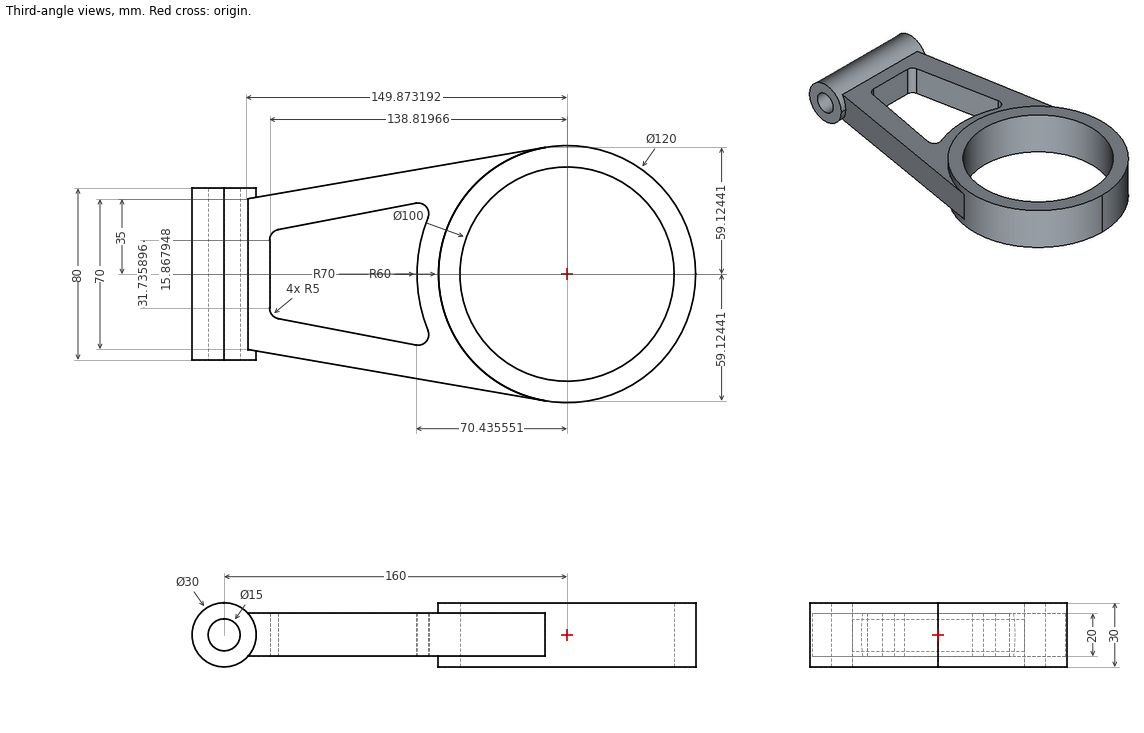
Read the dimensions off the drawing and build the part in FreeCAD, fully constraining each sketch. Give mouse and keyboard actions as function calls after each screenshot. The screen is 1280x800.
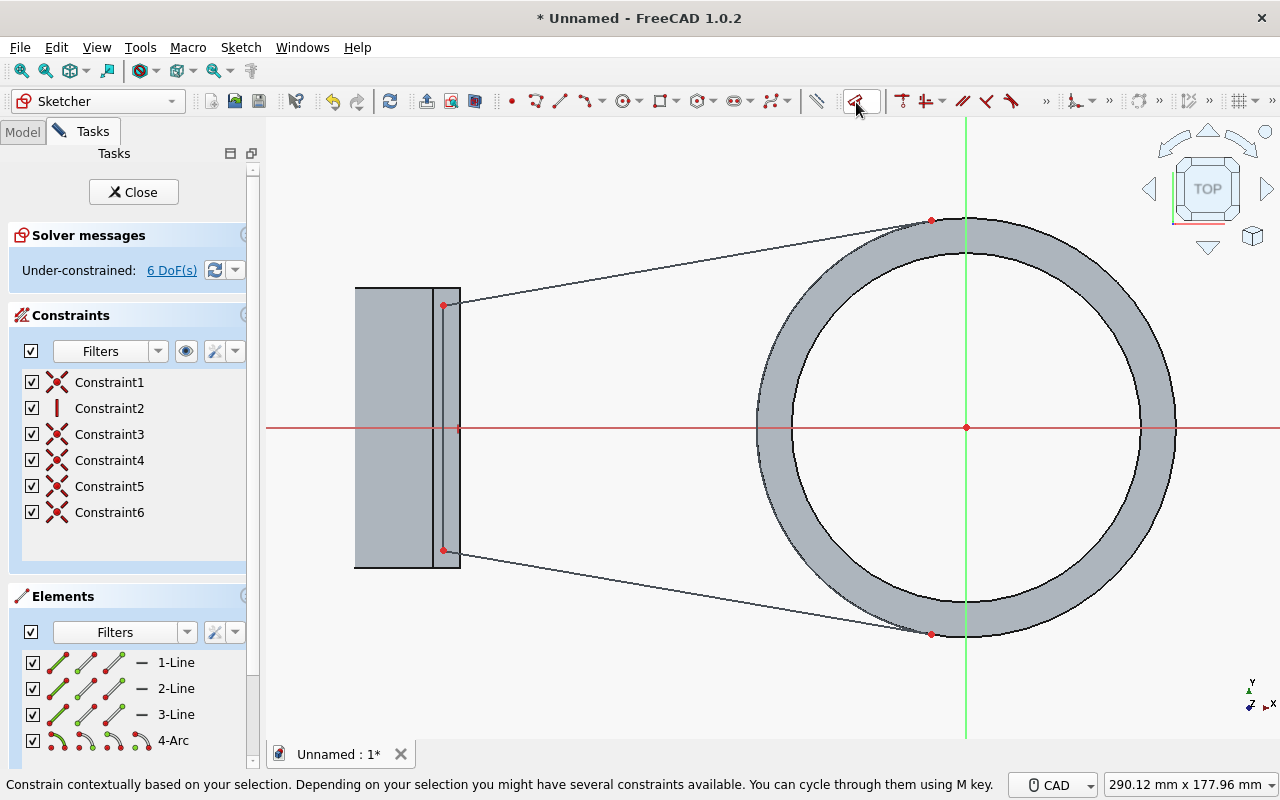
click(789, 316)
click(762, 299)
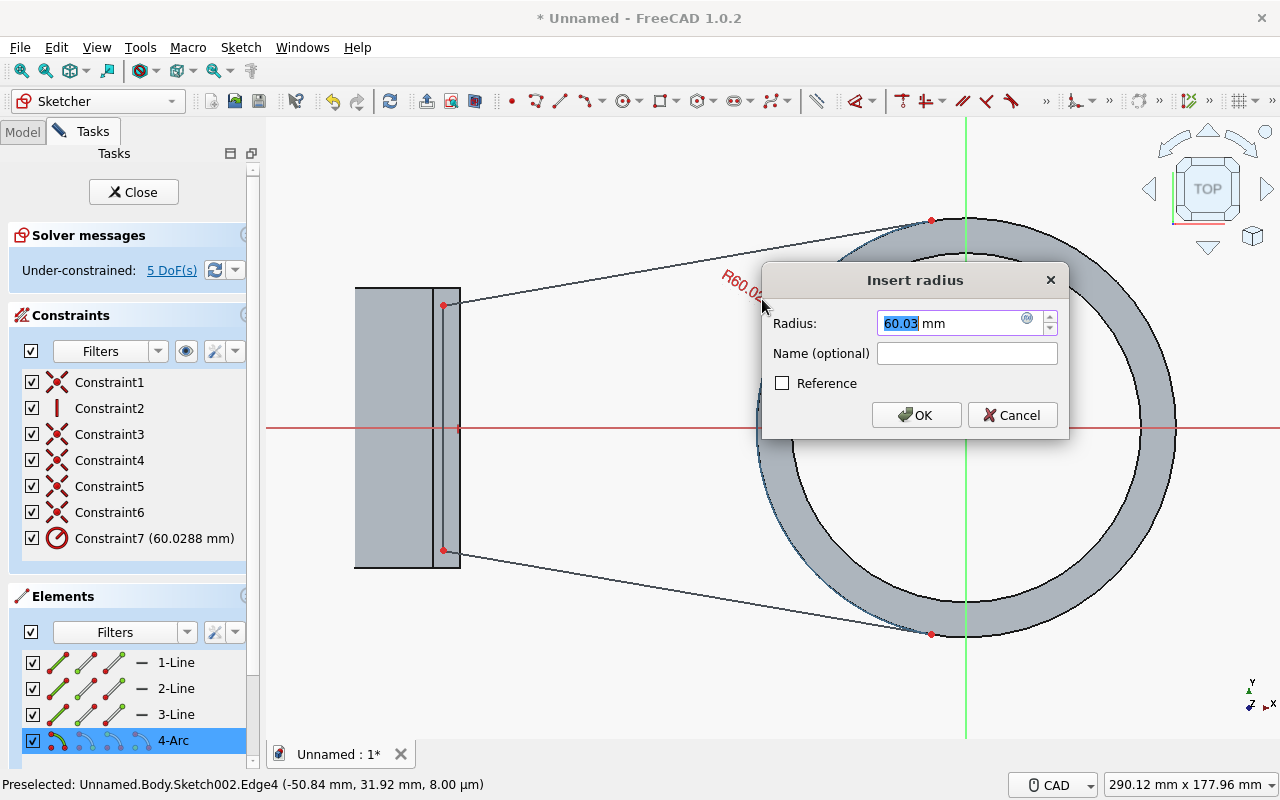
text(60)
key(Return)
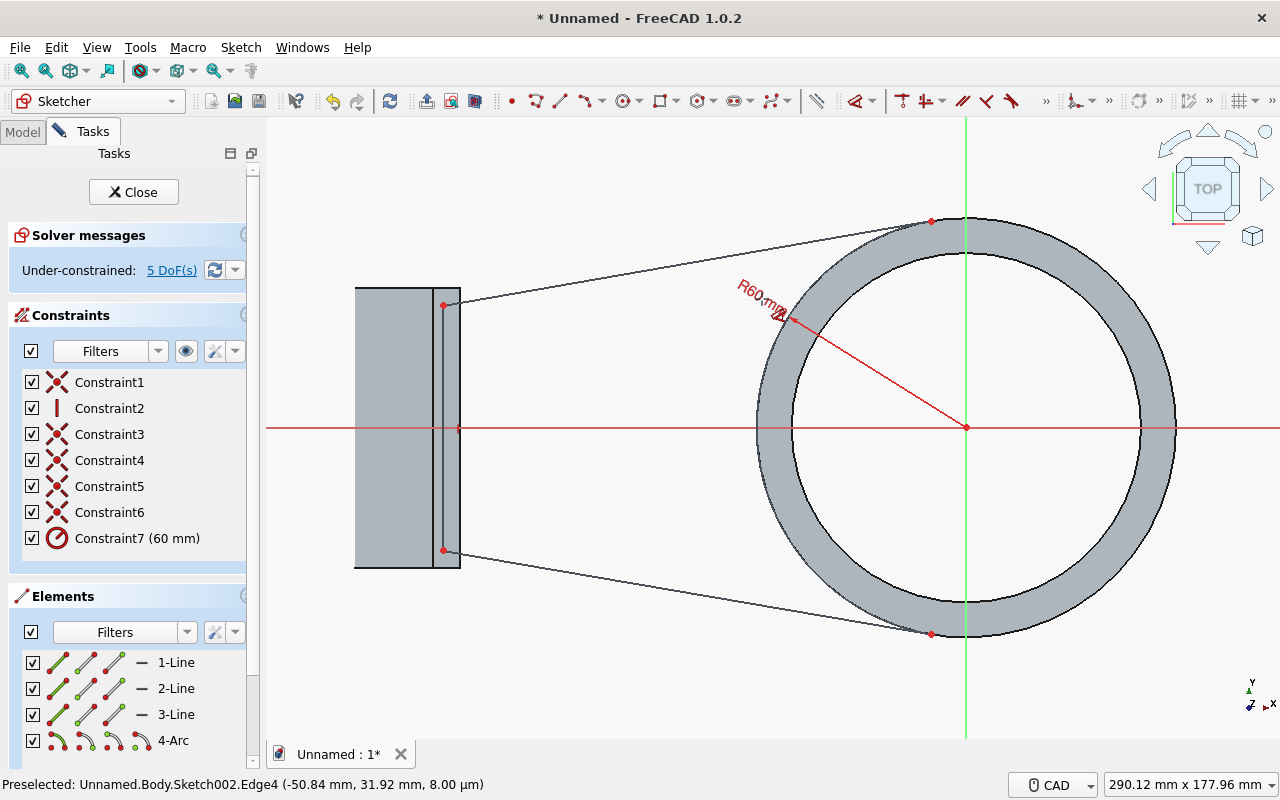
click(443, 380)
click(409, 372)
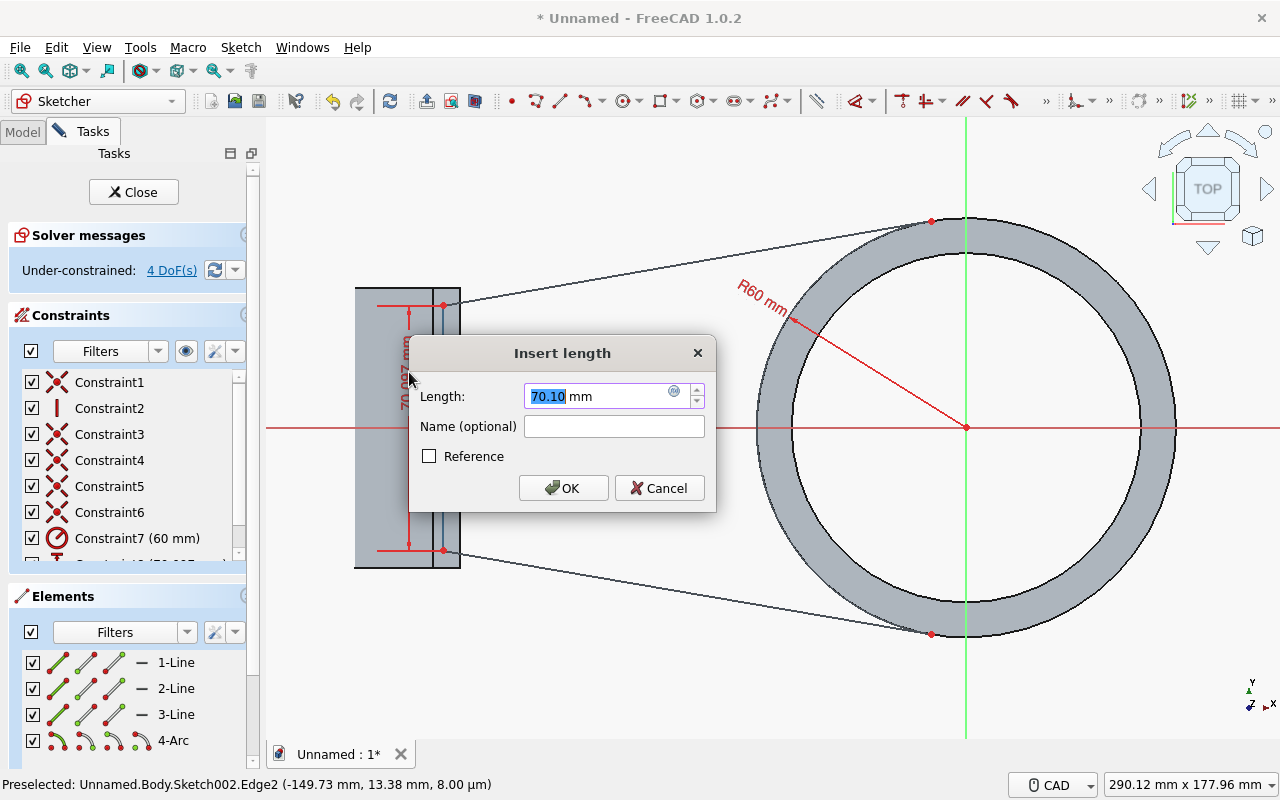
text(70)
key(Return)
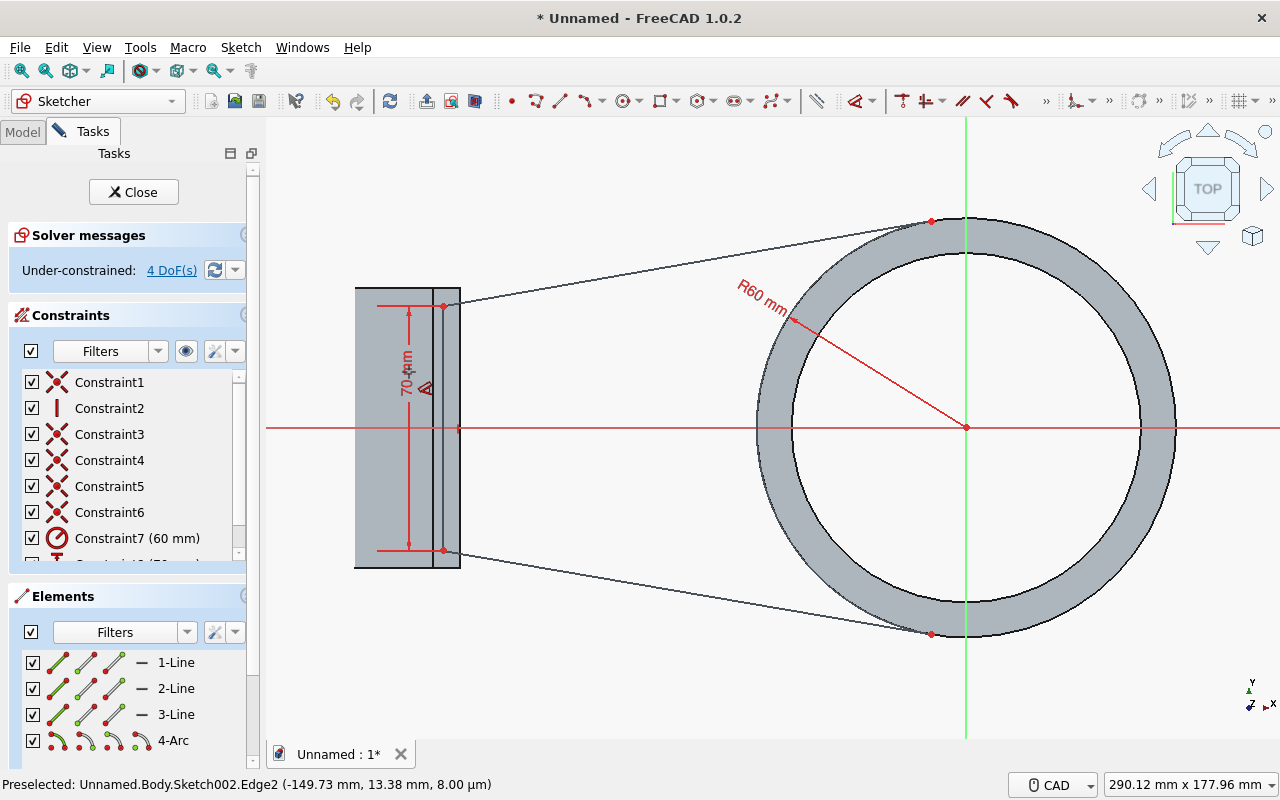
click(443, 306)
click(1000, 367)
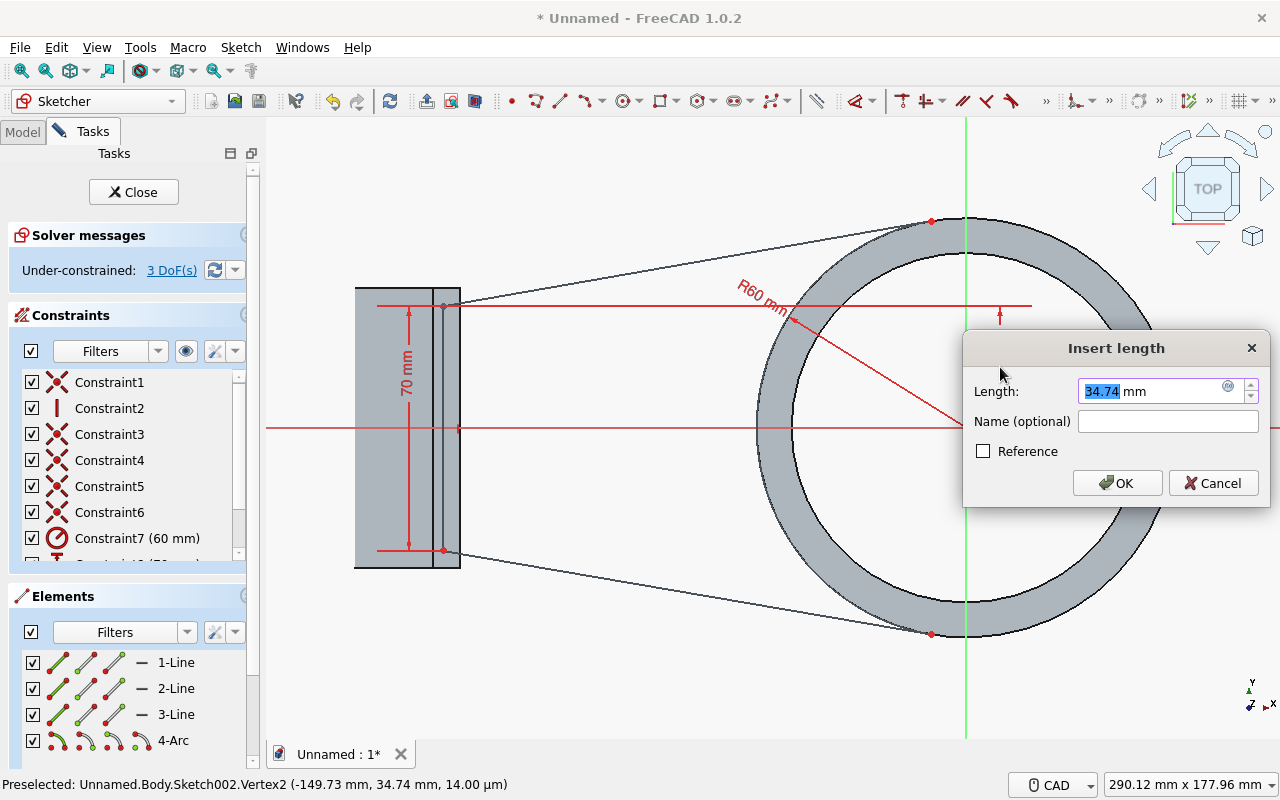
text(35)
key(Return)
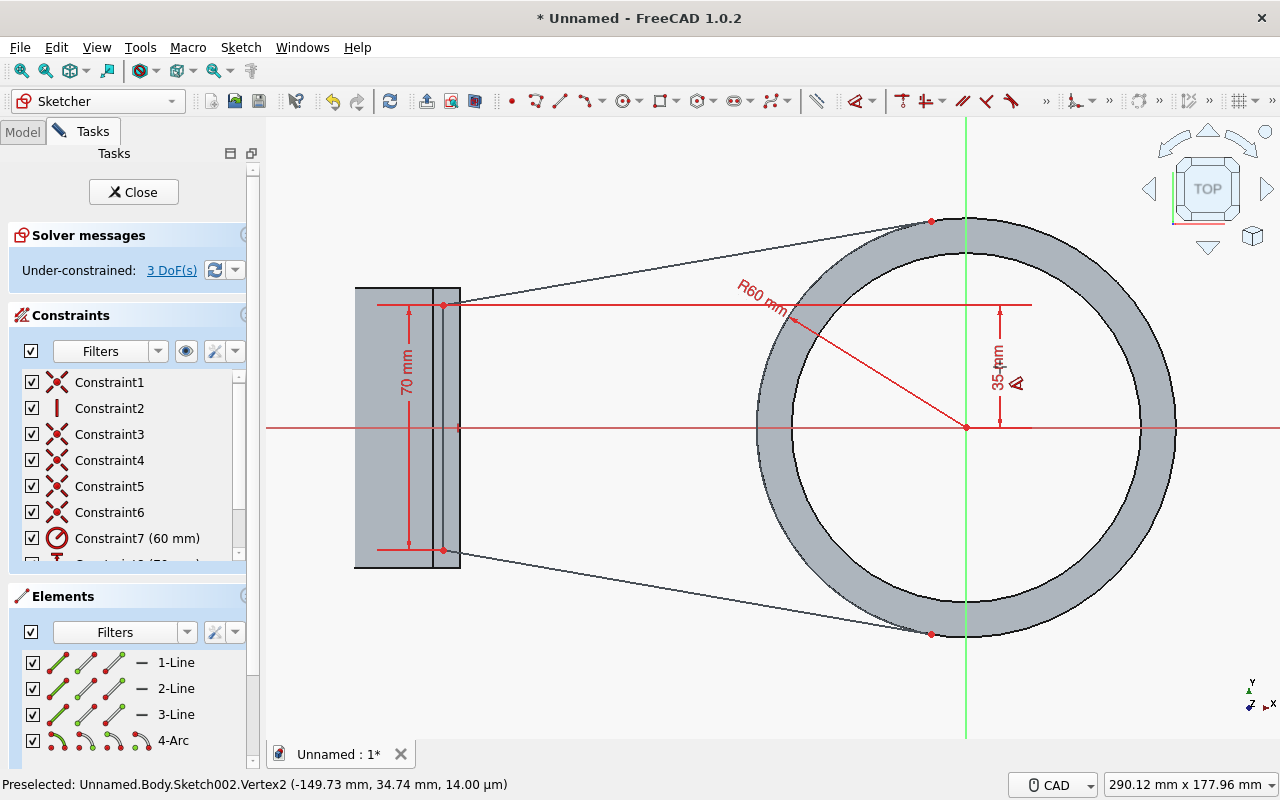
click(931, 221)
click(1000, 324)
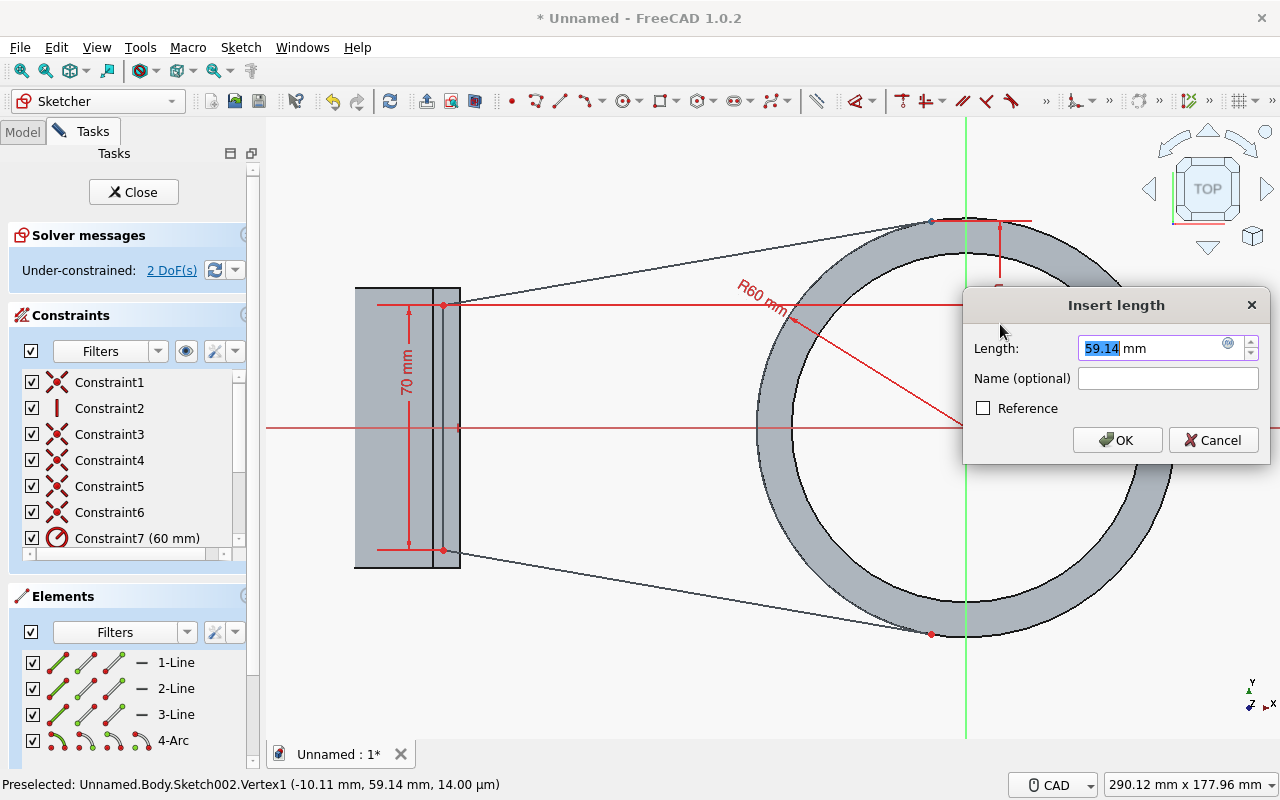
text(59.12441)
key(Return)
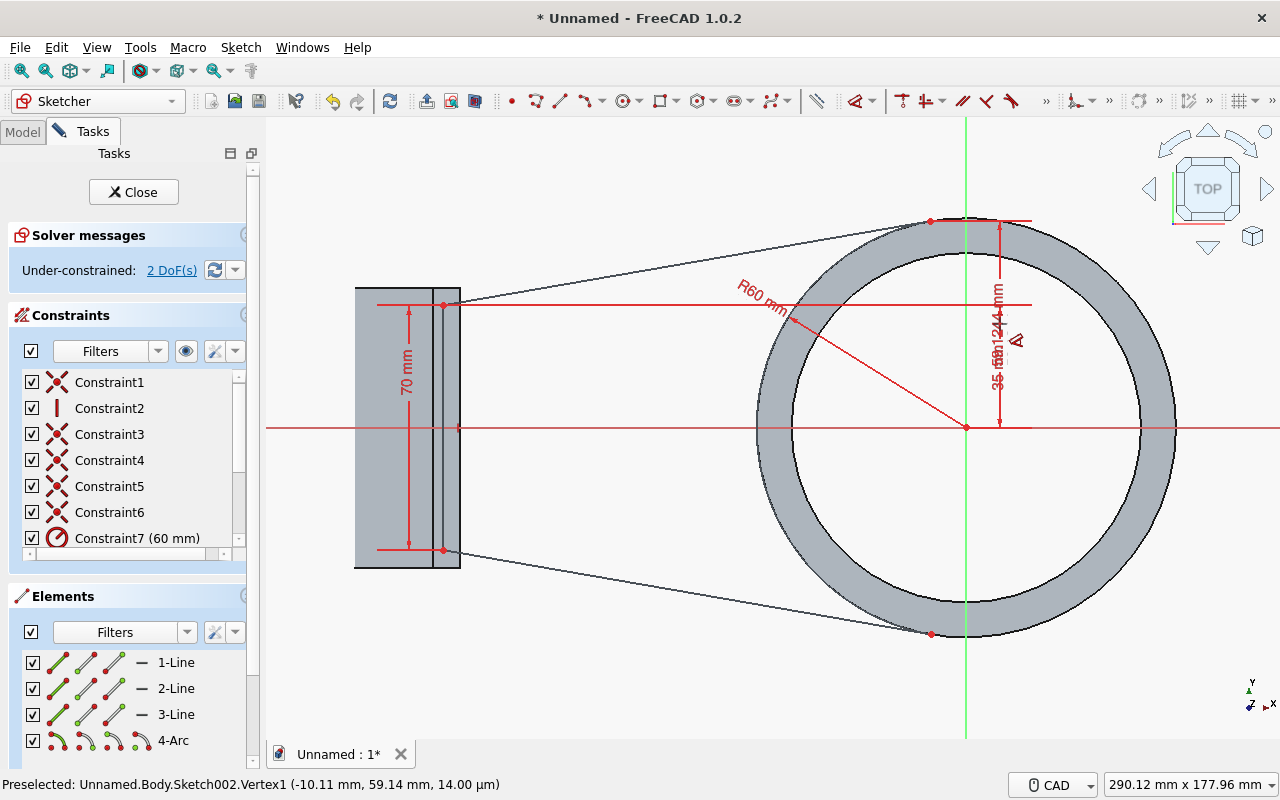
click(931, 634)
click(1000, 531)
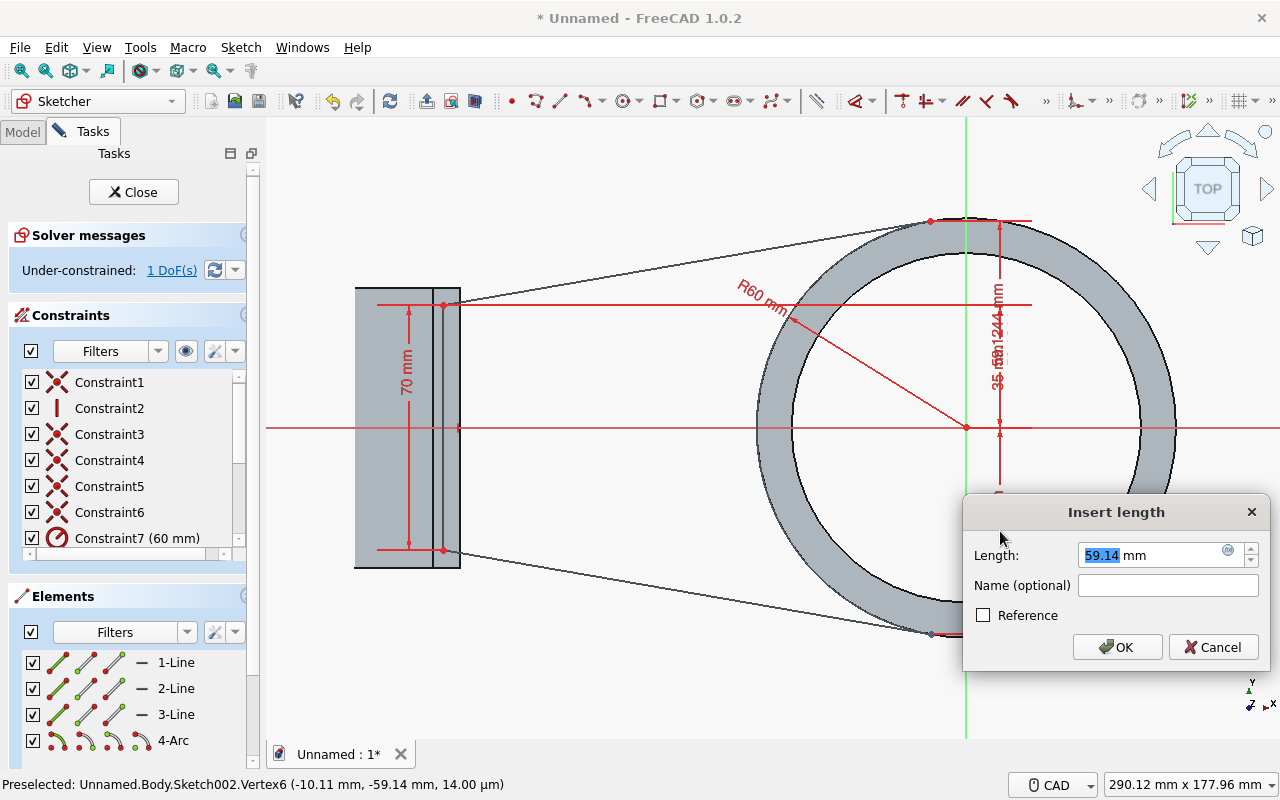
text(59.12441)
key(Return)